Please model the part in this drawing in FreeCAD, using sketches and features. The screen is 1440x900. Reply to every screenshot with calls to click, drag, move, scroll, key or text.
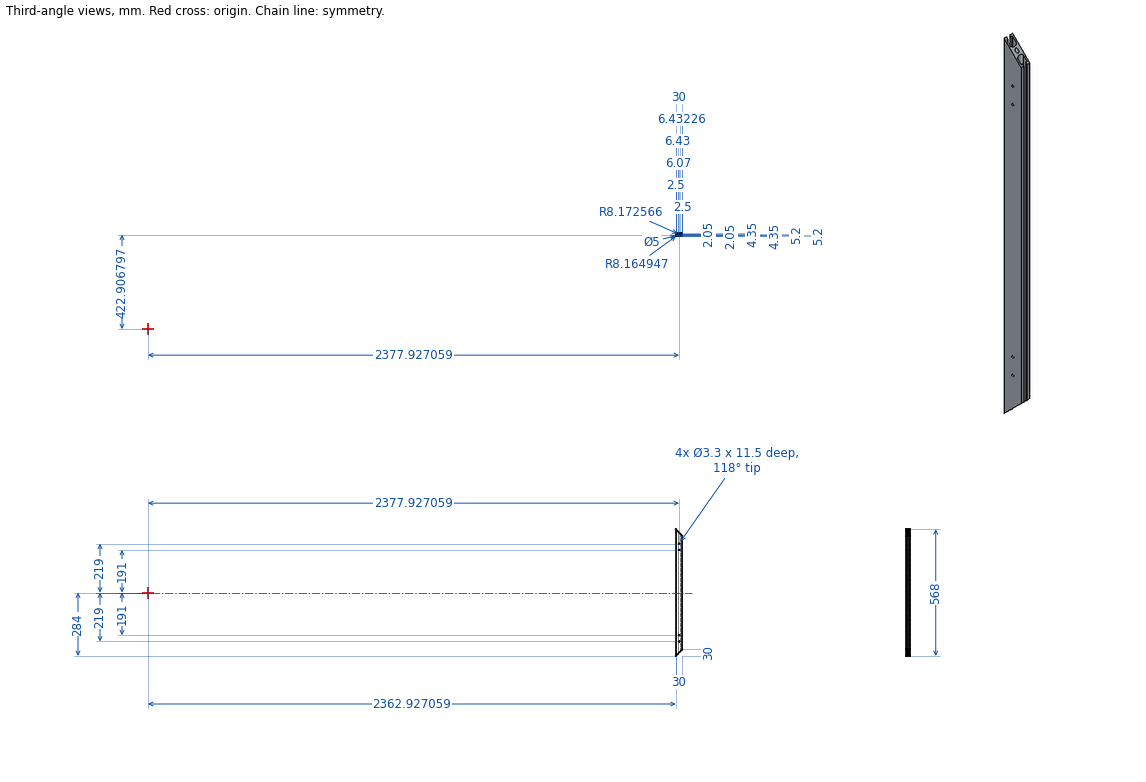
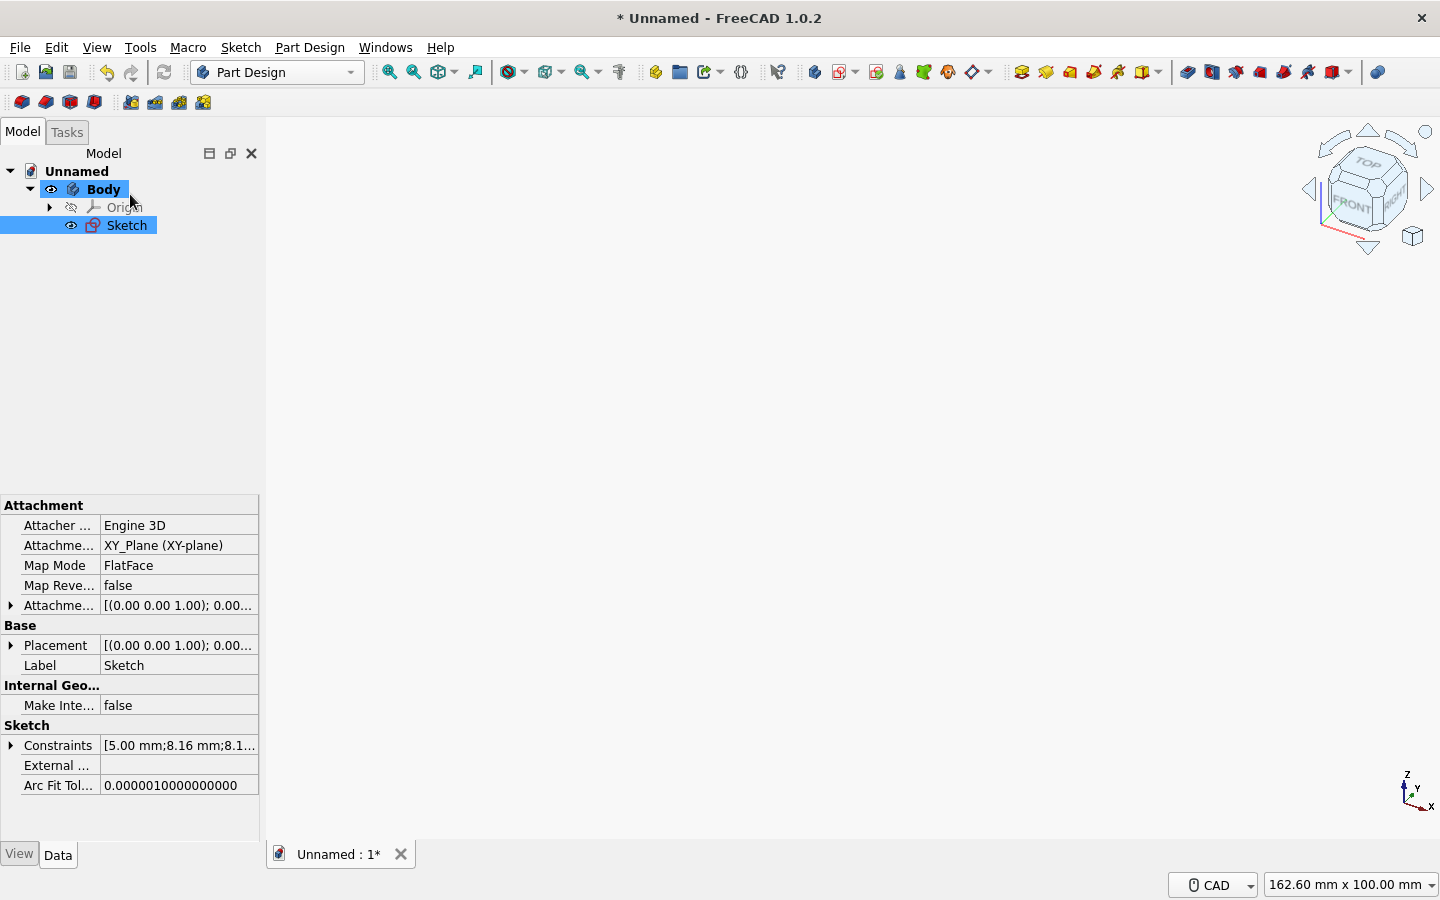
click(1022, 72)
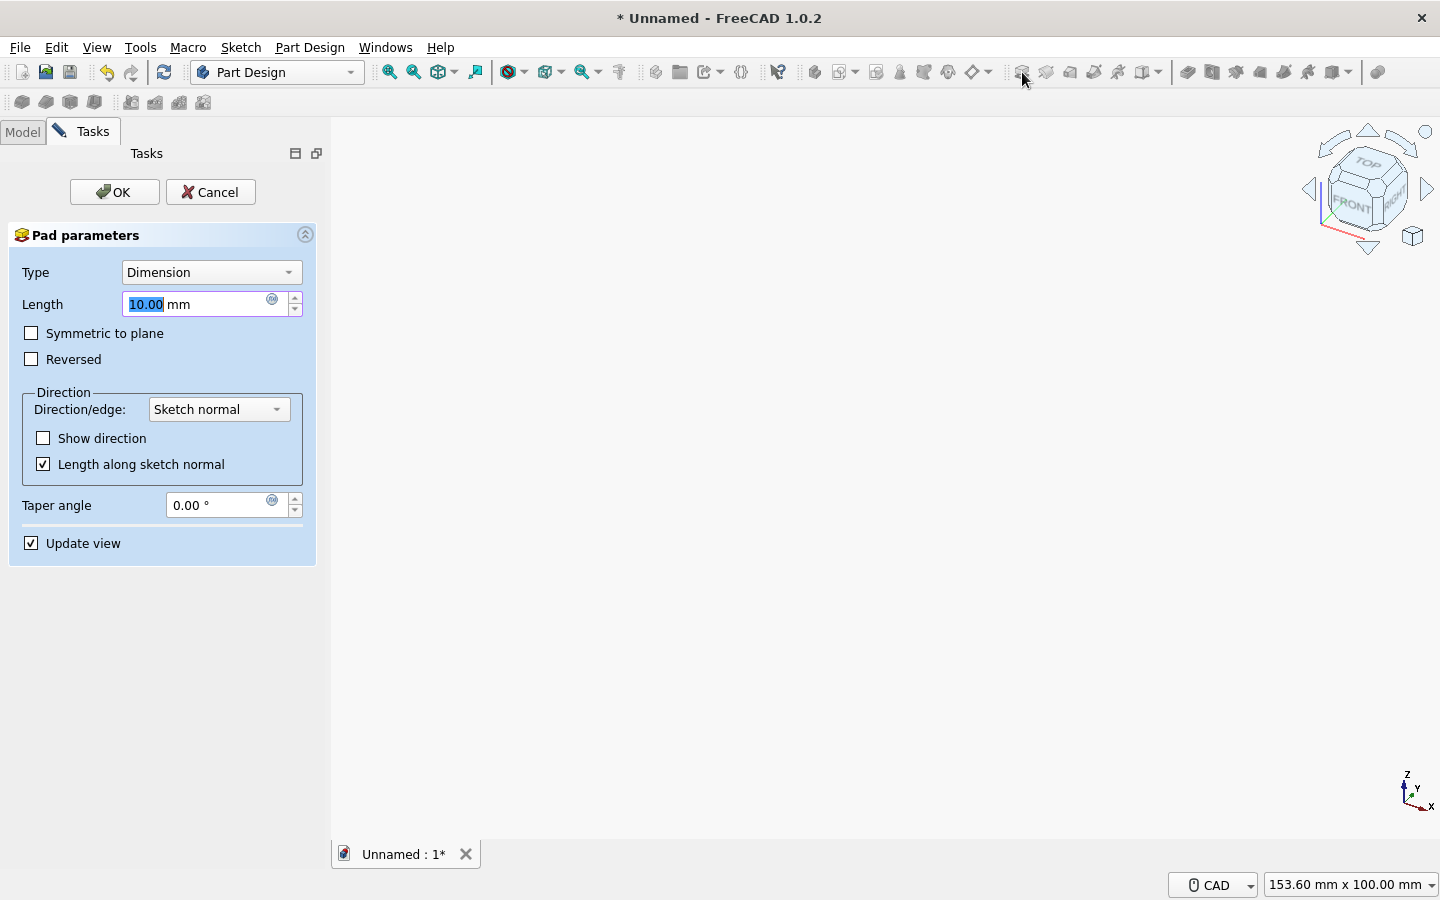
text(568)
key(Tab)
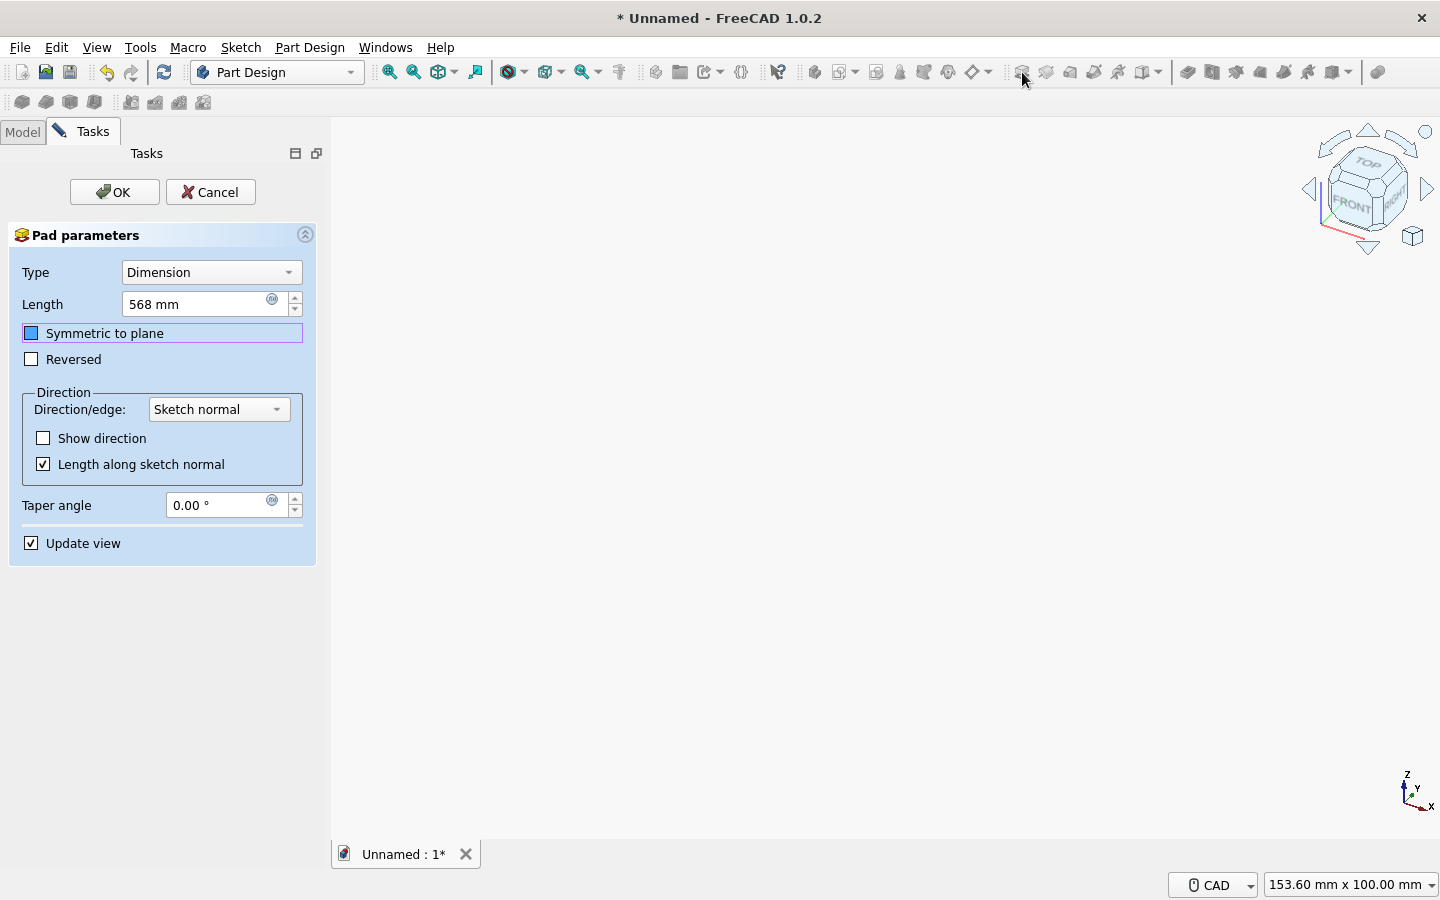
click(30, 333)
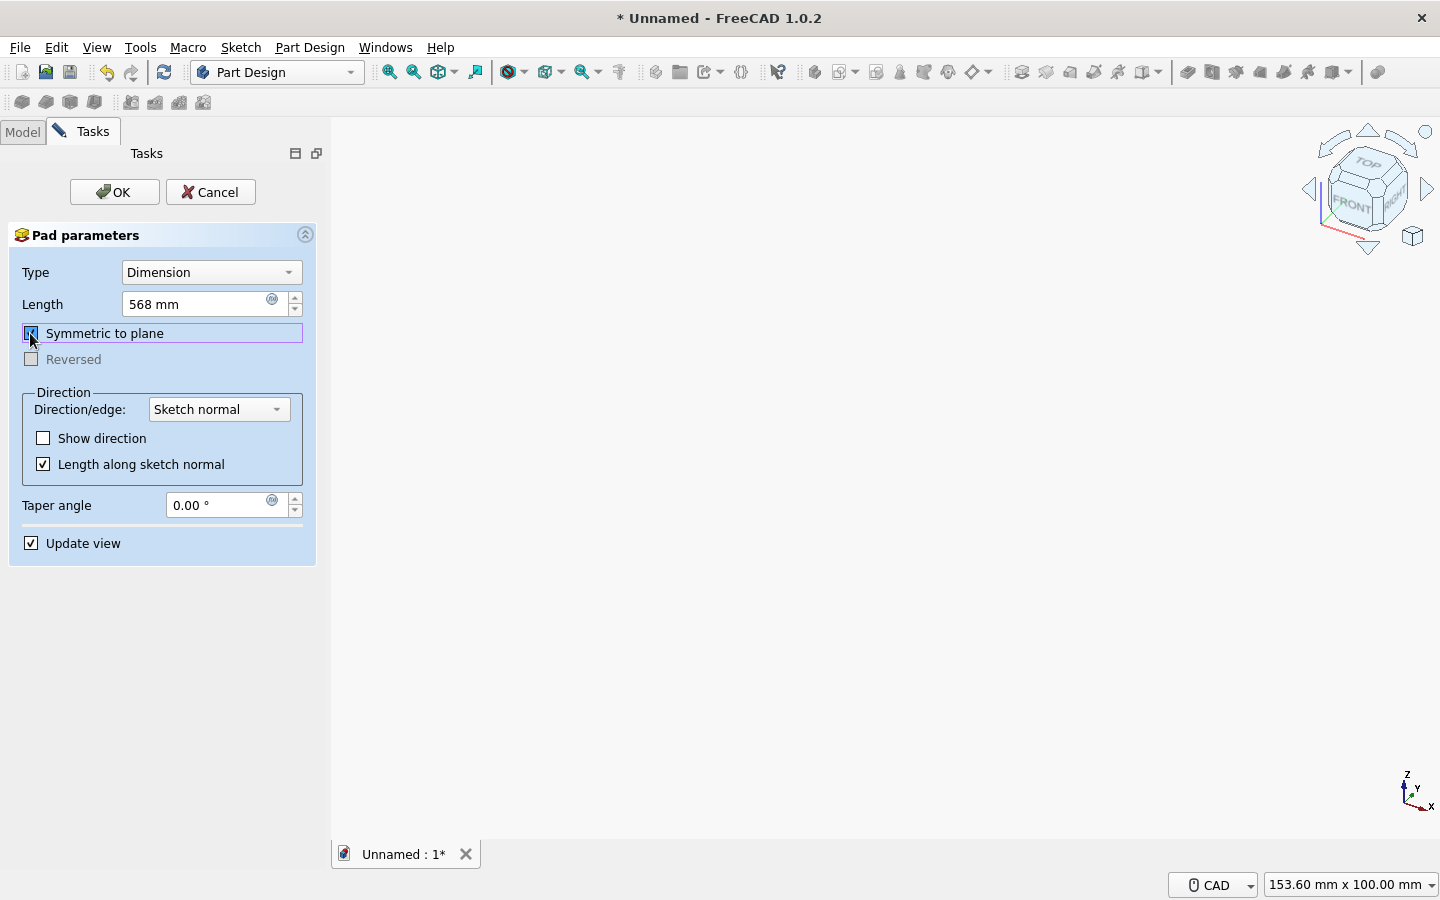
click(115, 192)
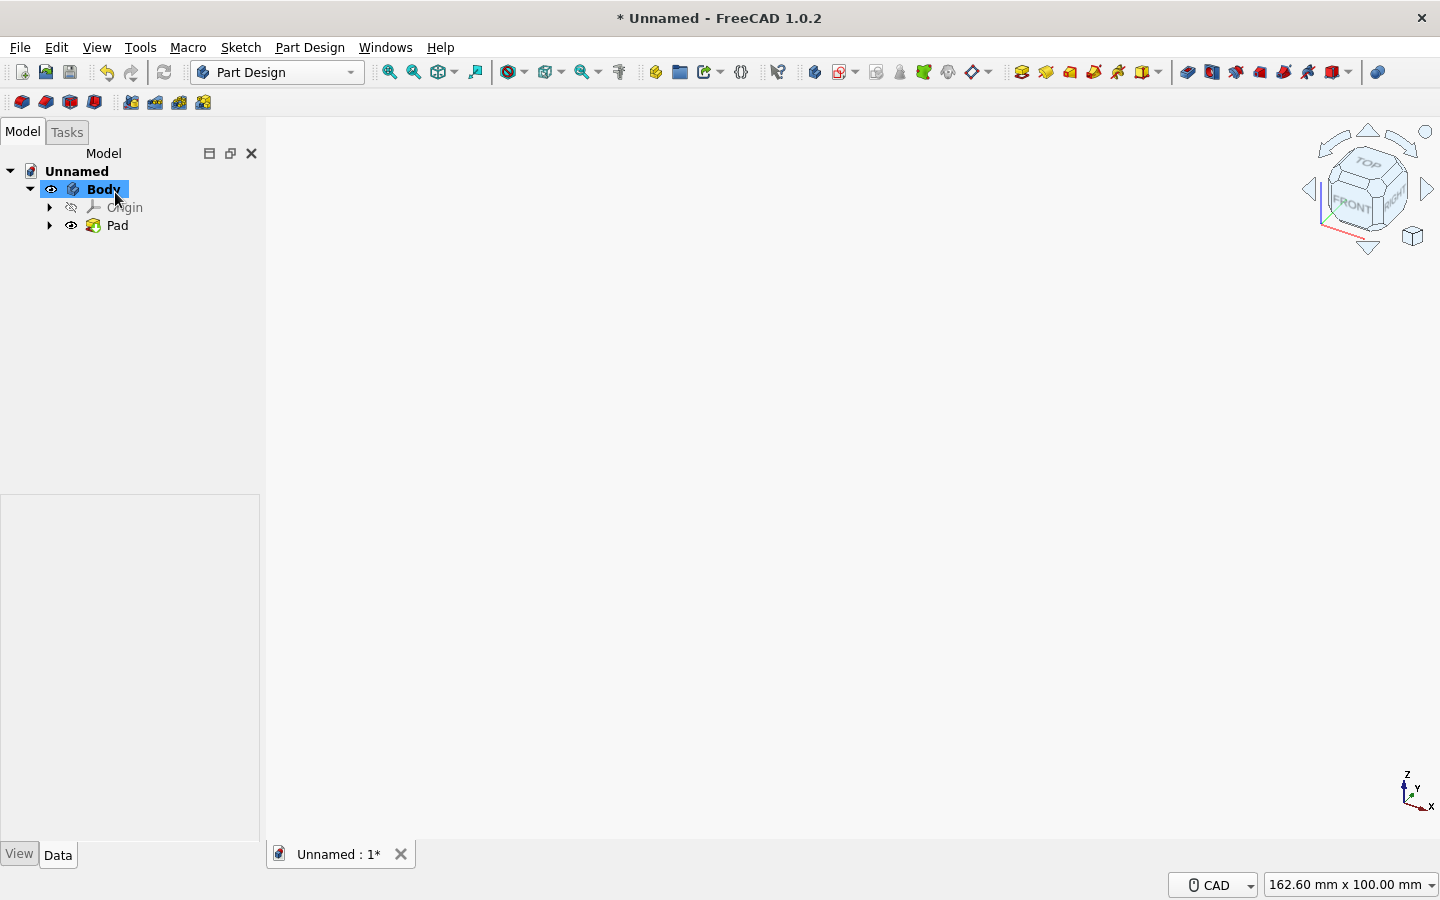
click(390, 72)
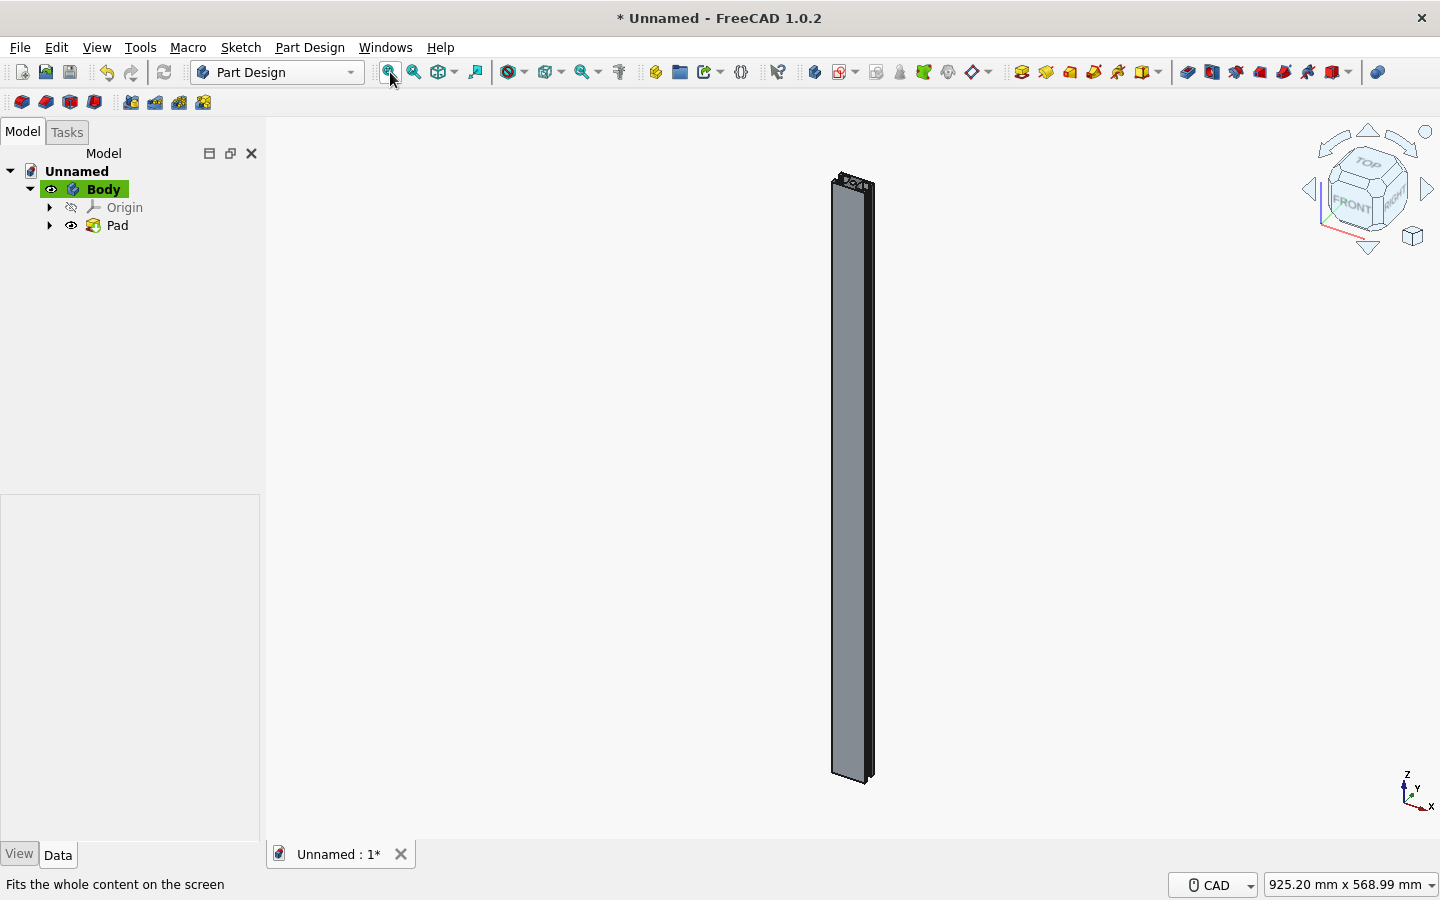
key(4)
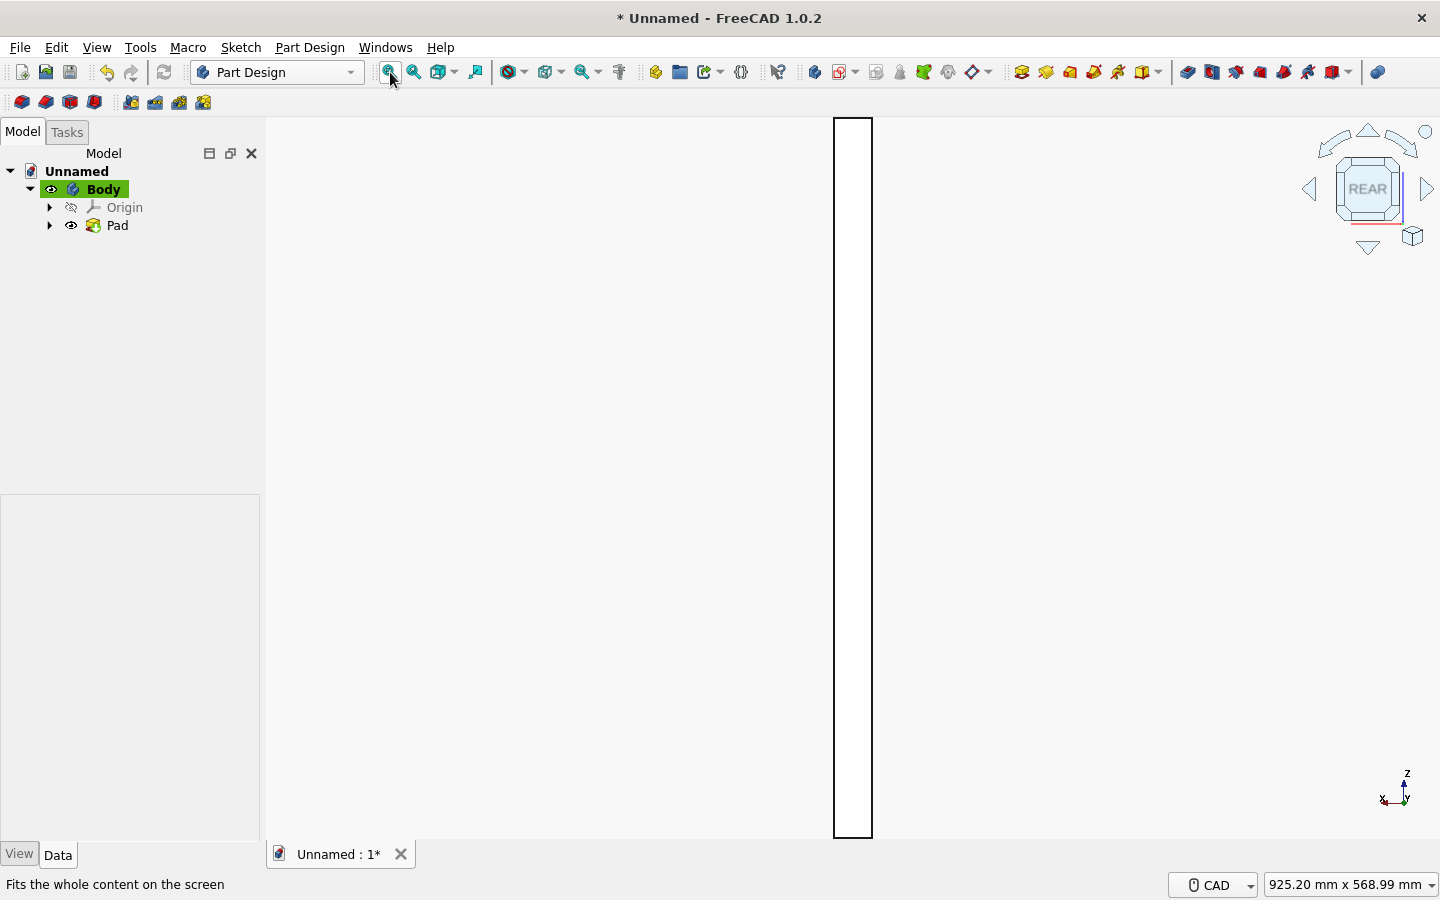
click(853, 168)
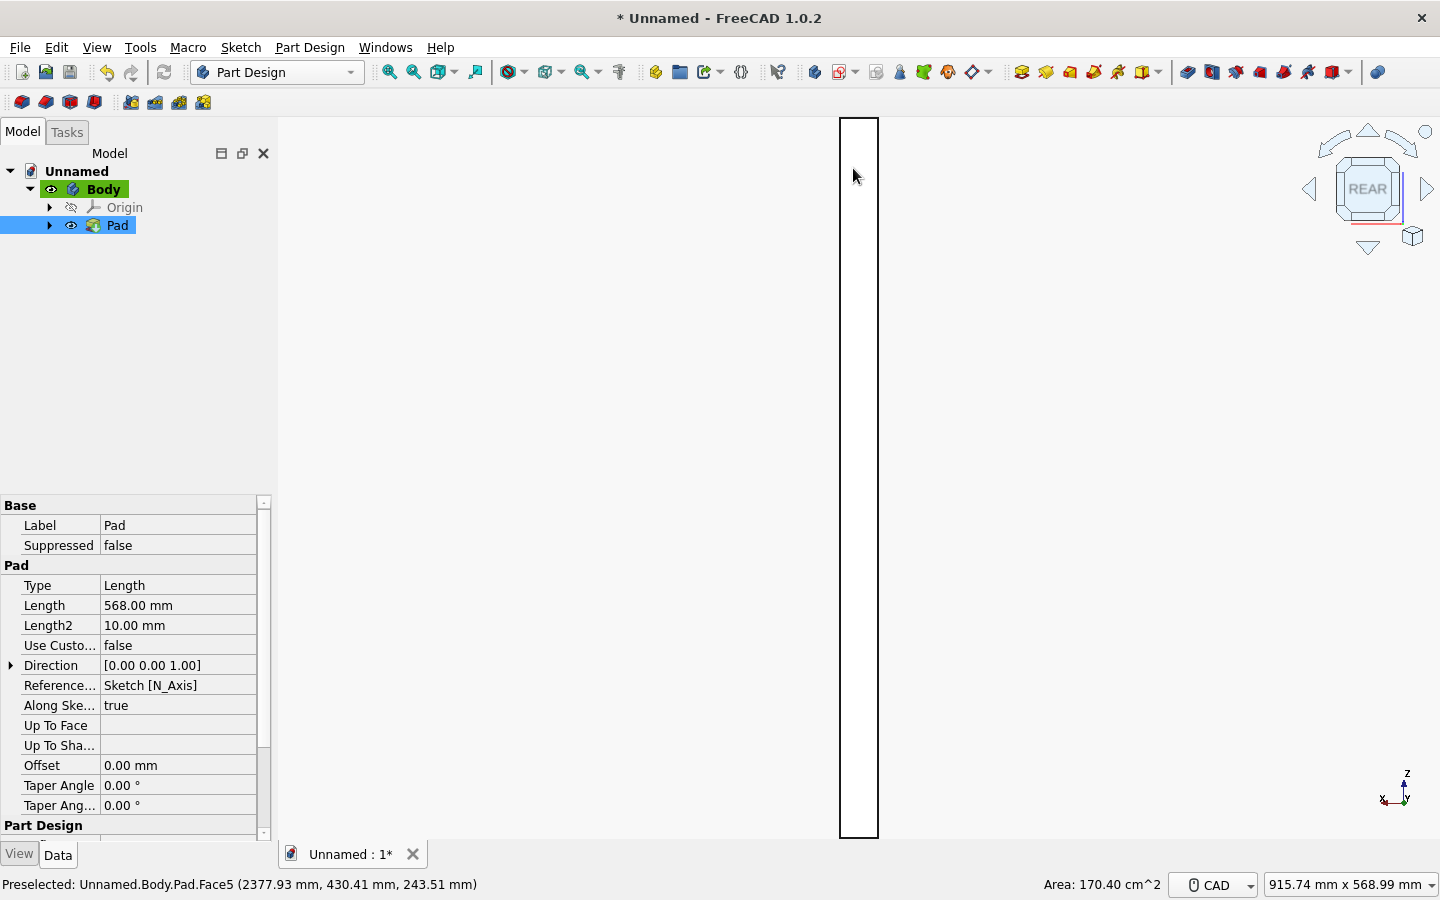
click(840, 72)